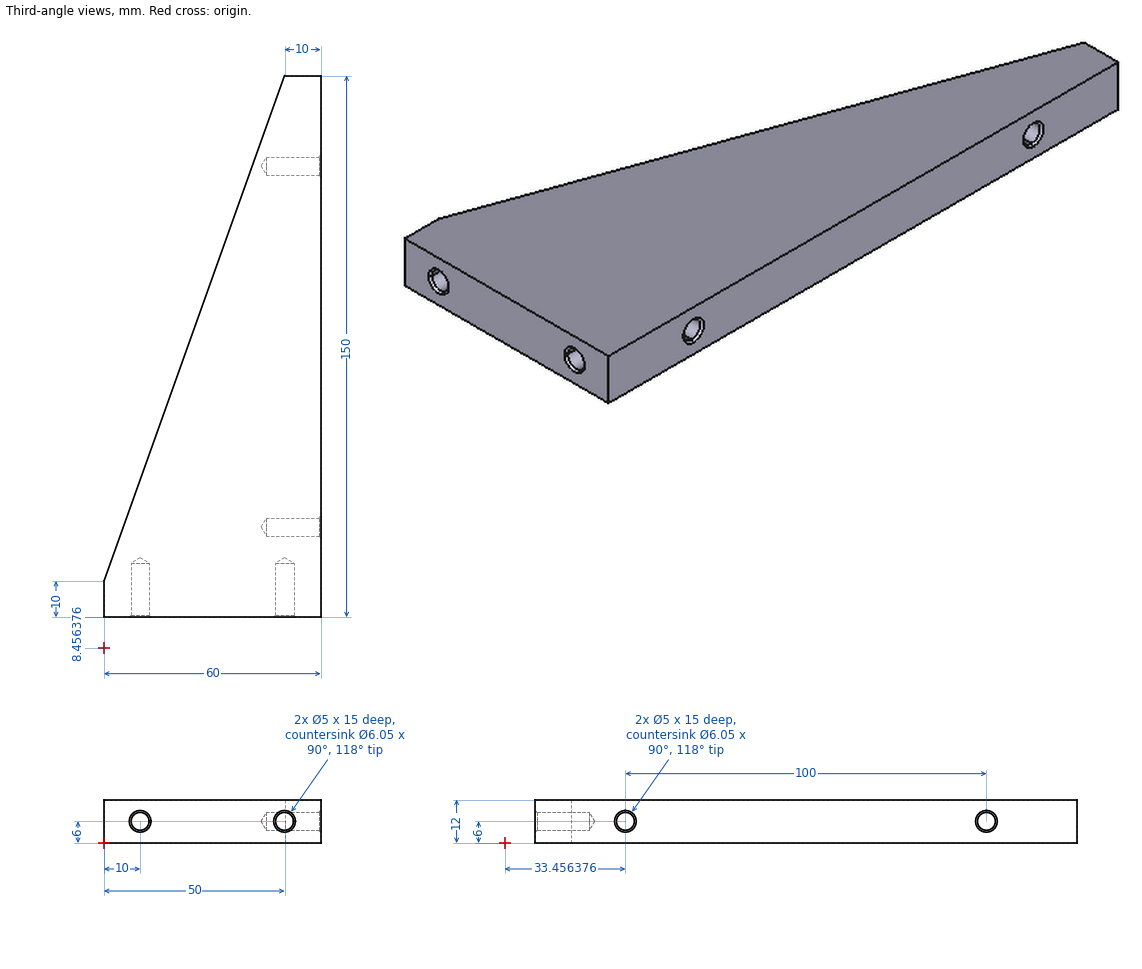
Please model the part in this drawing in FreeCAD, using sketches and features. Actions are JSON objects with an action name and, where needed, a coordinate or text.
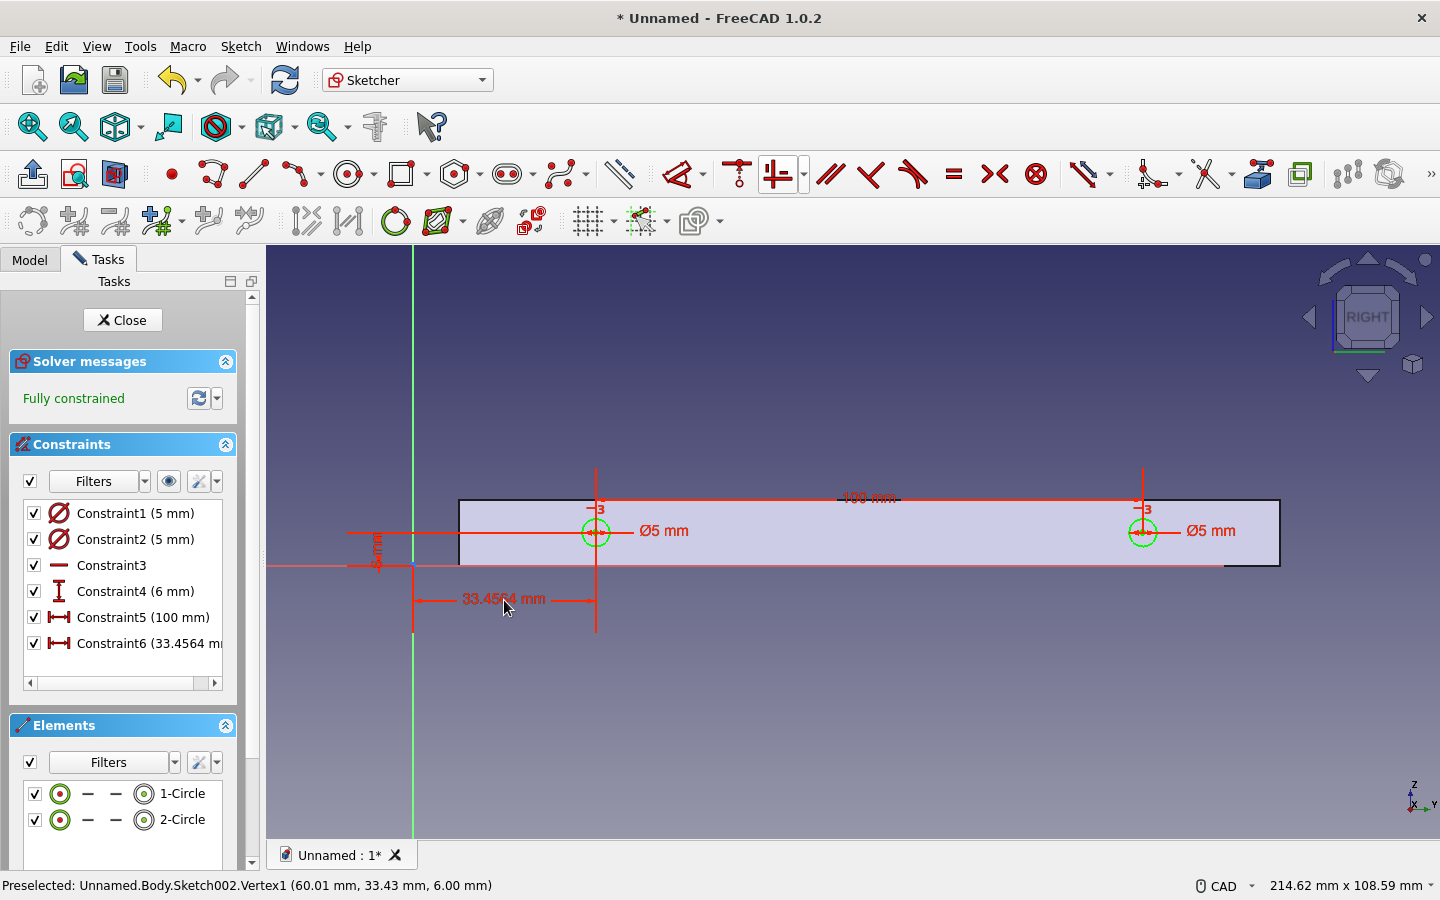
{"action": "left_click", "coordinate": [123, 320]}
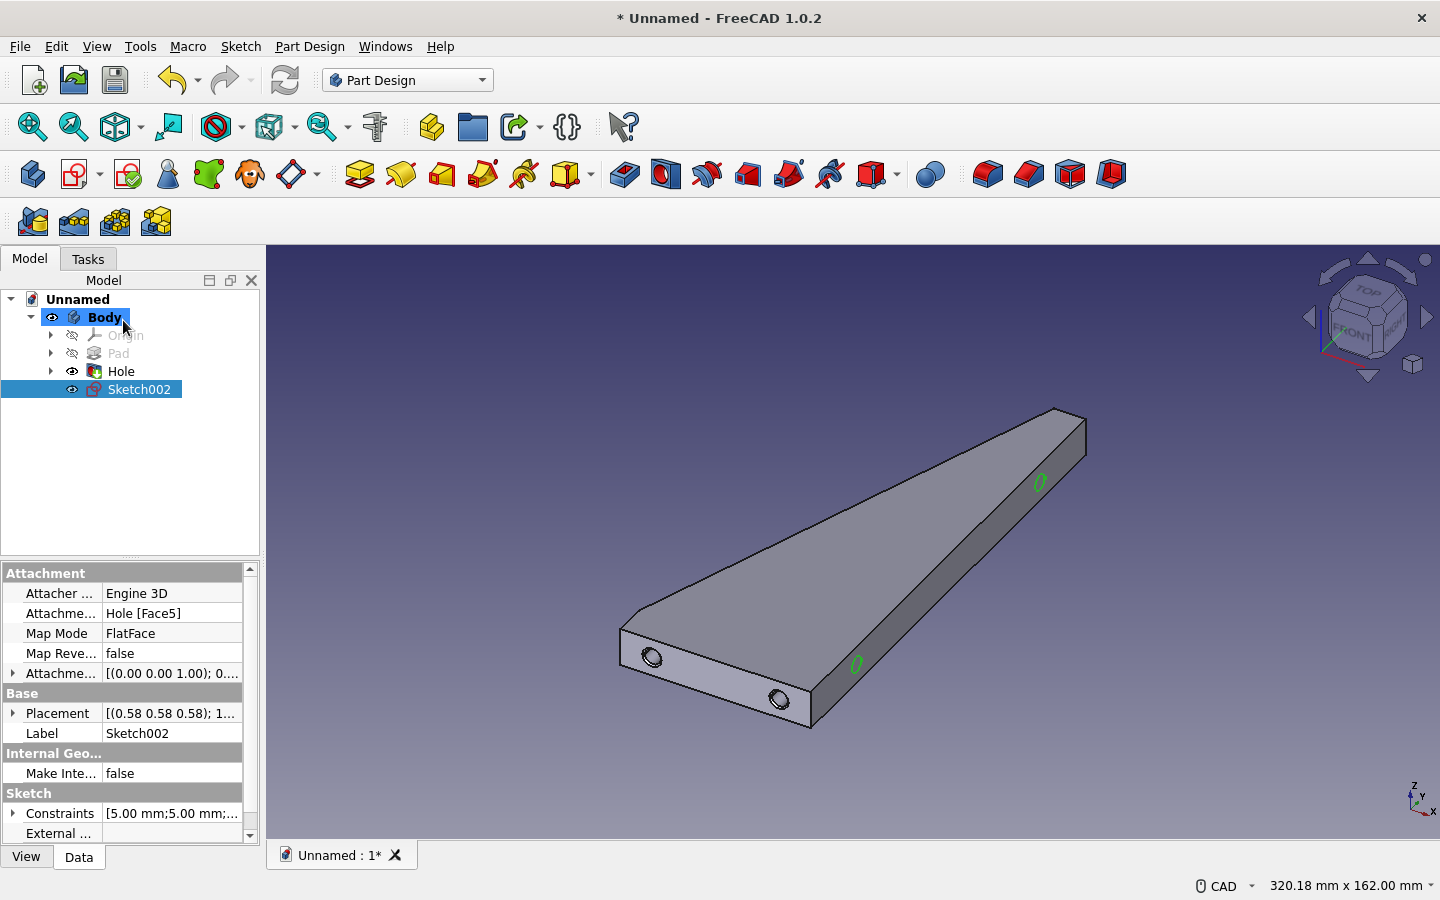
{"action": "left_click", "coordinate": [666, 174]}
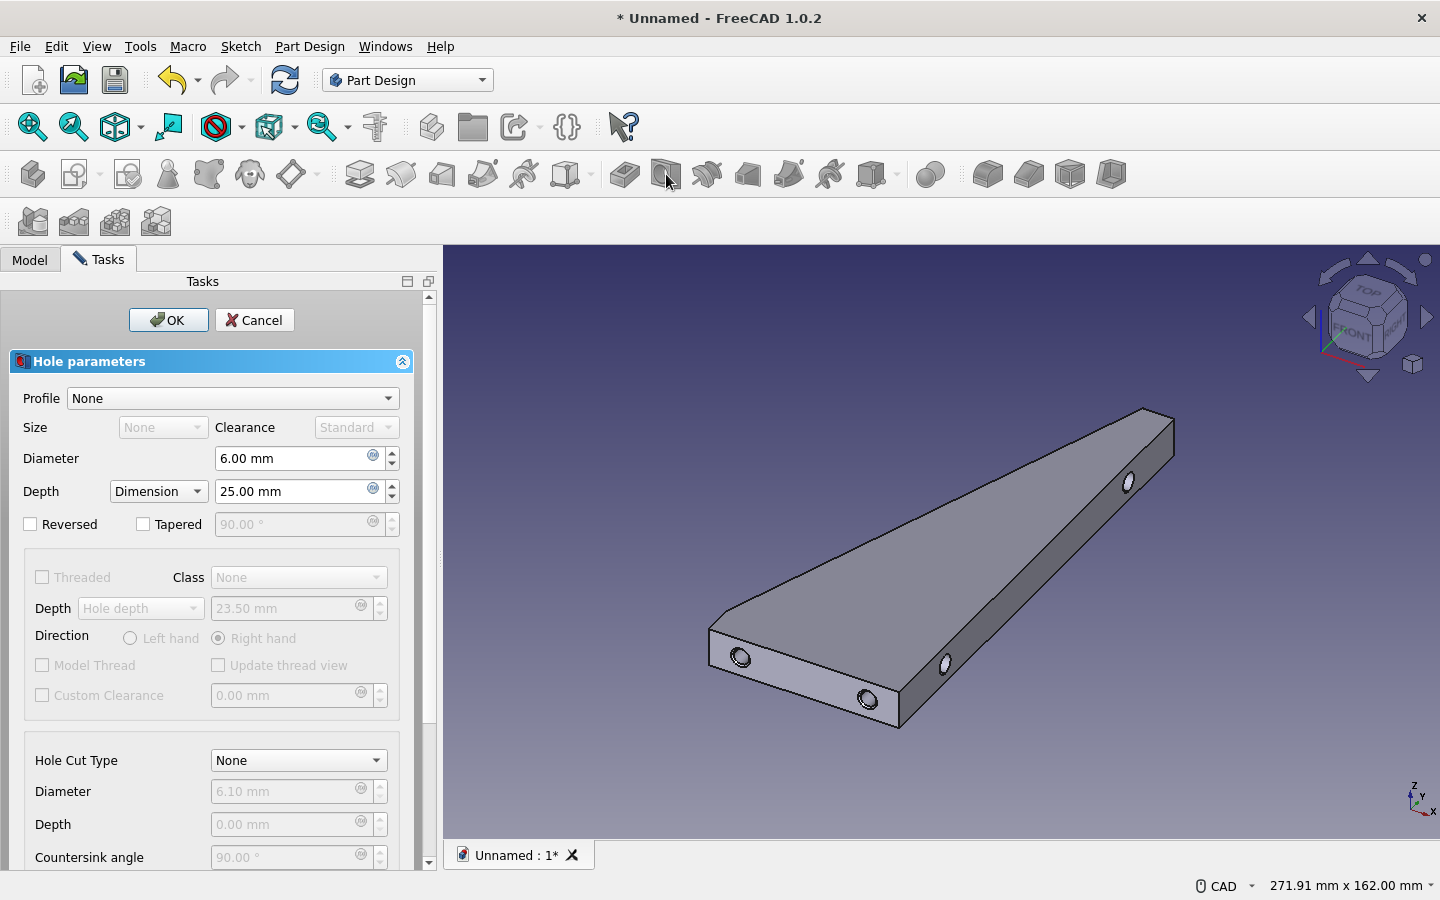
{"action": "triple_click", "coordinate": [300, 458]}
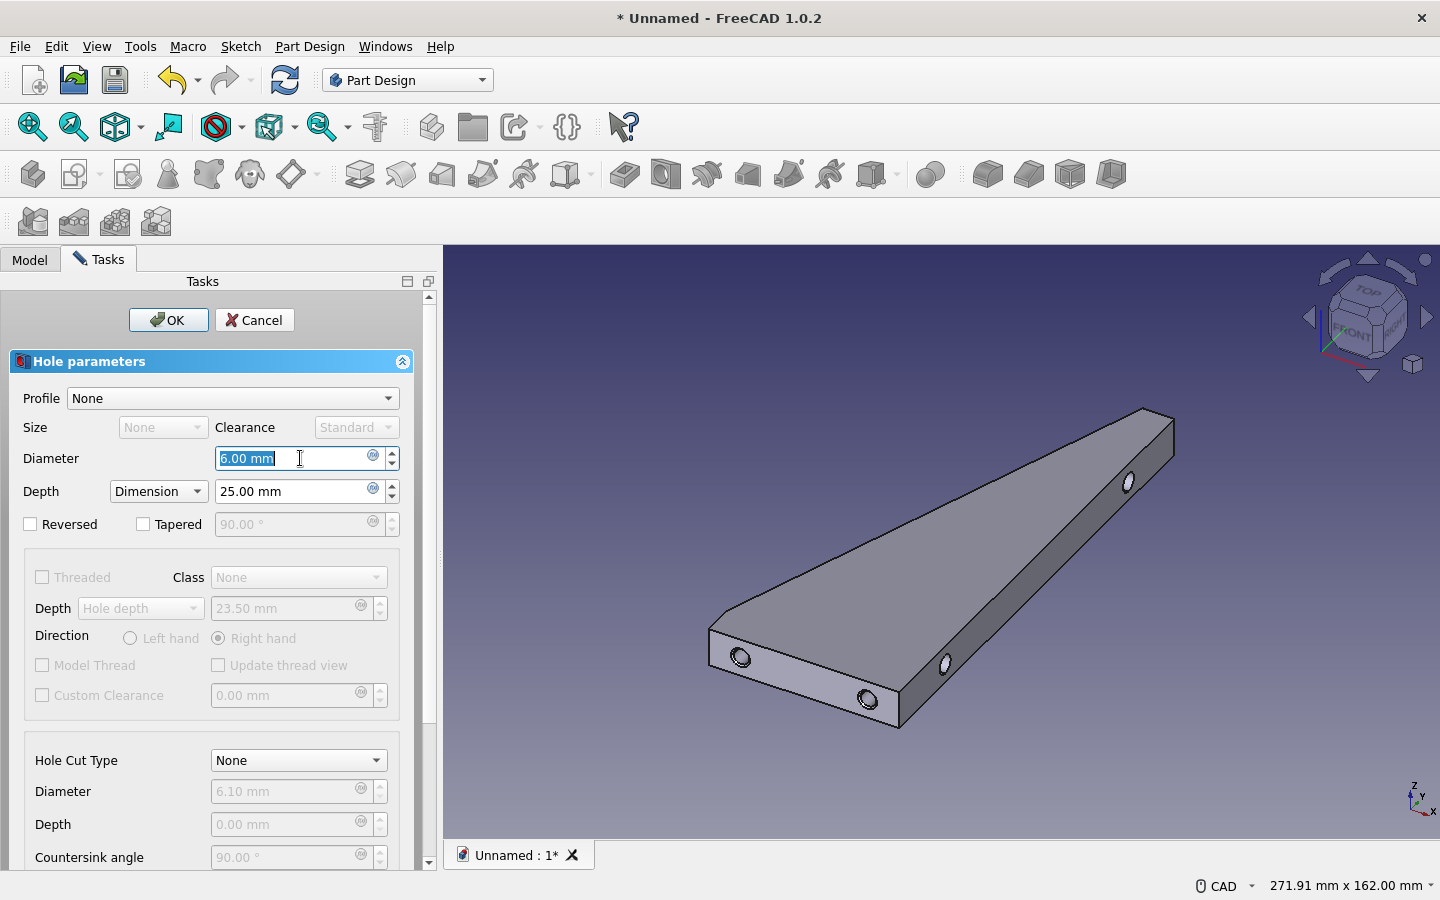
{"action": "type", "text": "5"}
{"action": "key", "text": "Tab"}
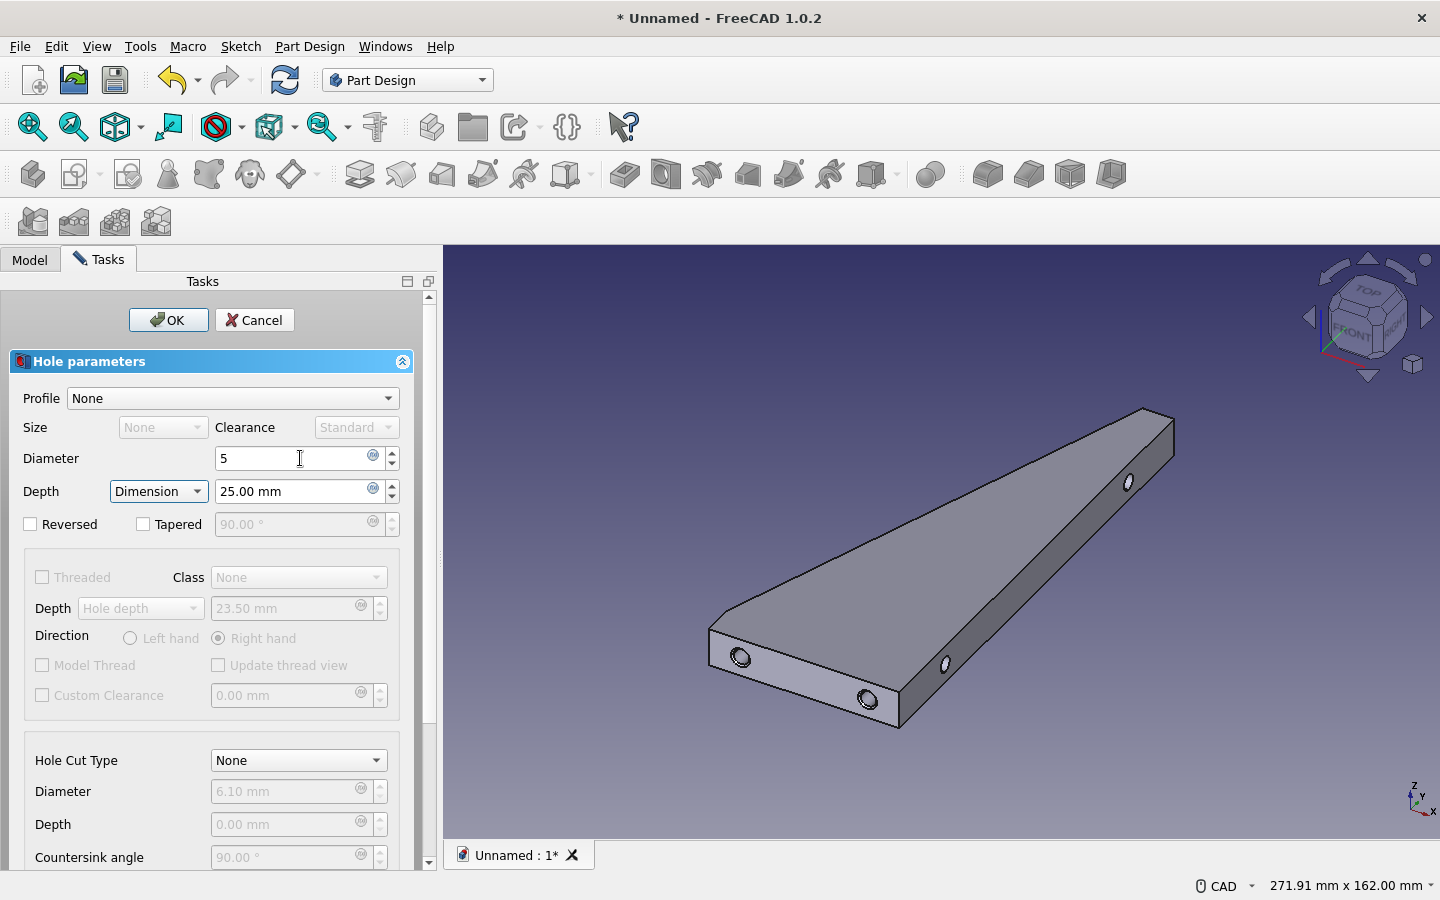
{"action": "triple_click", "coordinate": [300, 492]}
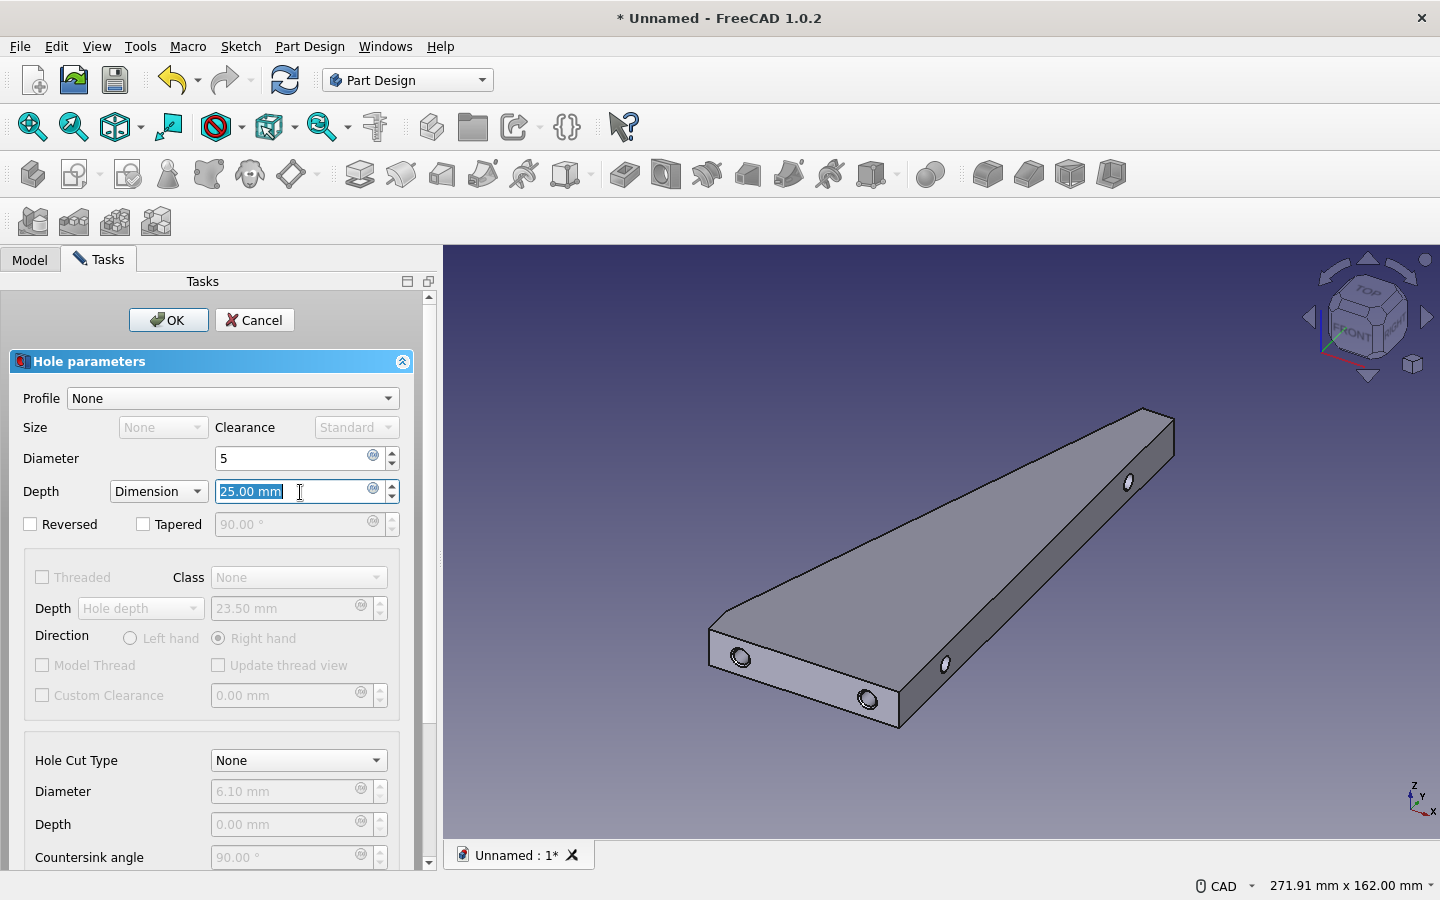
{"action": "type", "text": "15"}
{"action": "key", "text": "Tab"}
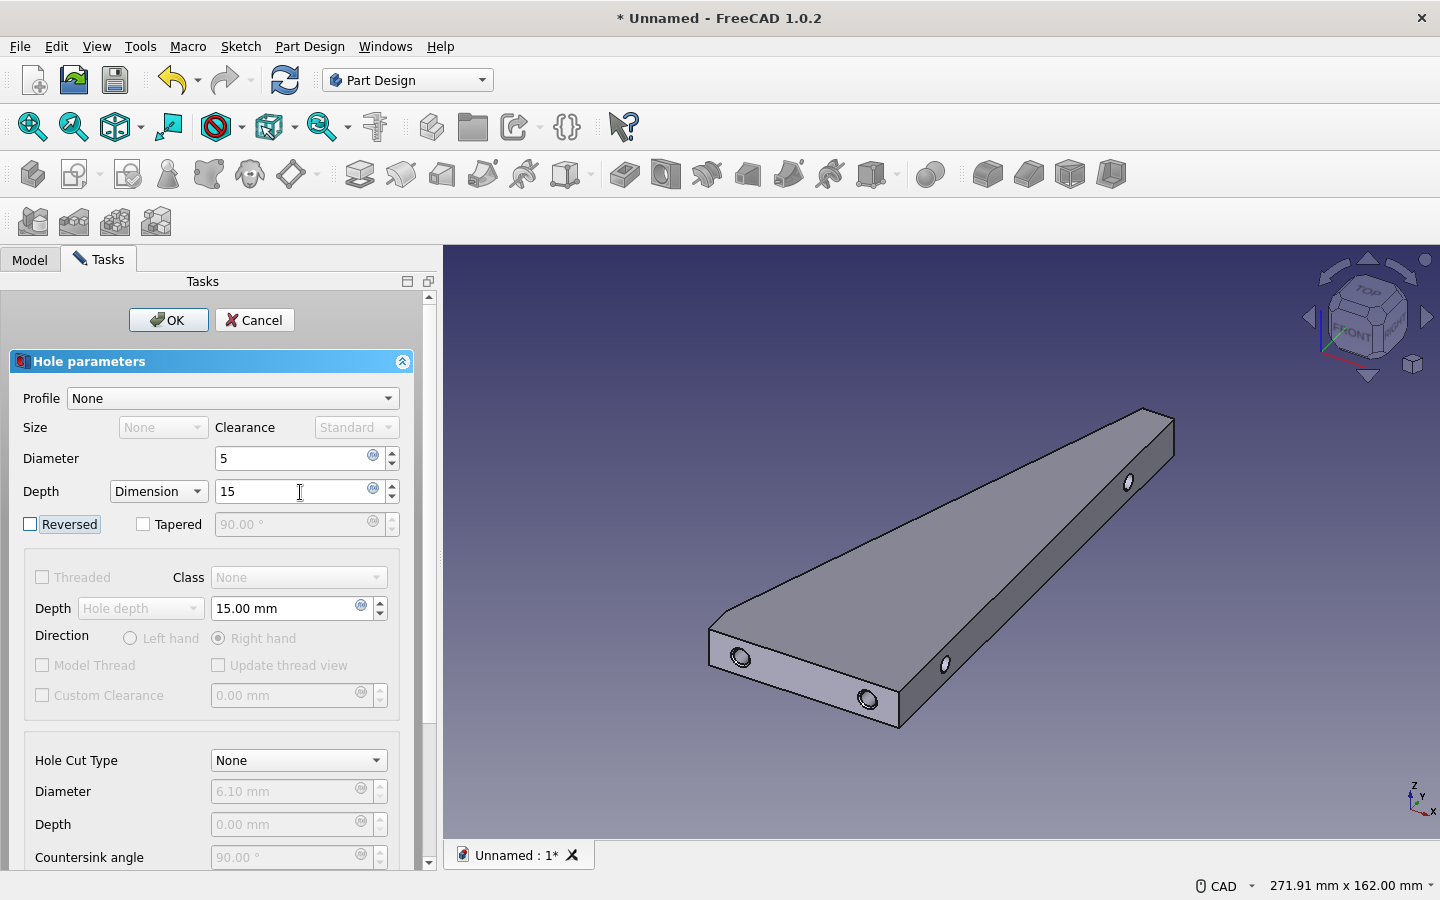
{"action": "left_click", "coordinate": [300, 760]}